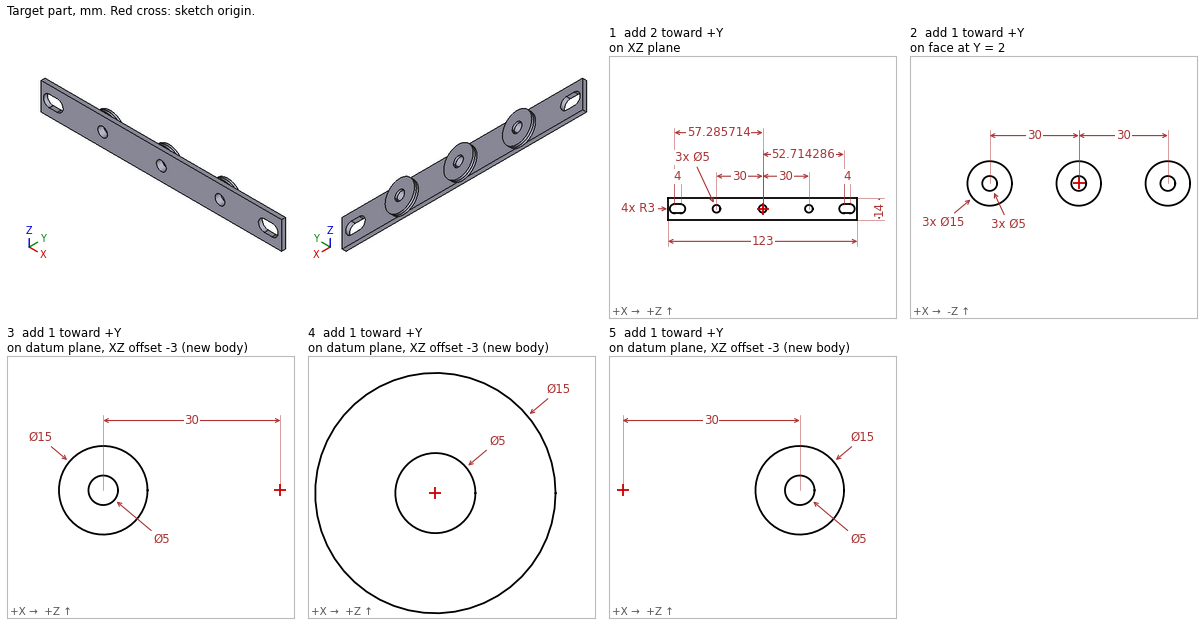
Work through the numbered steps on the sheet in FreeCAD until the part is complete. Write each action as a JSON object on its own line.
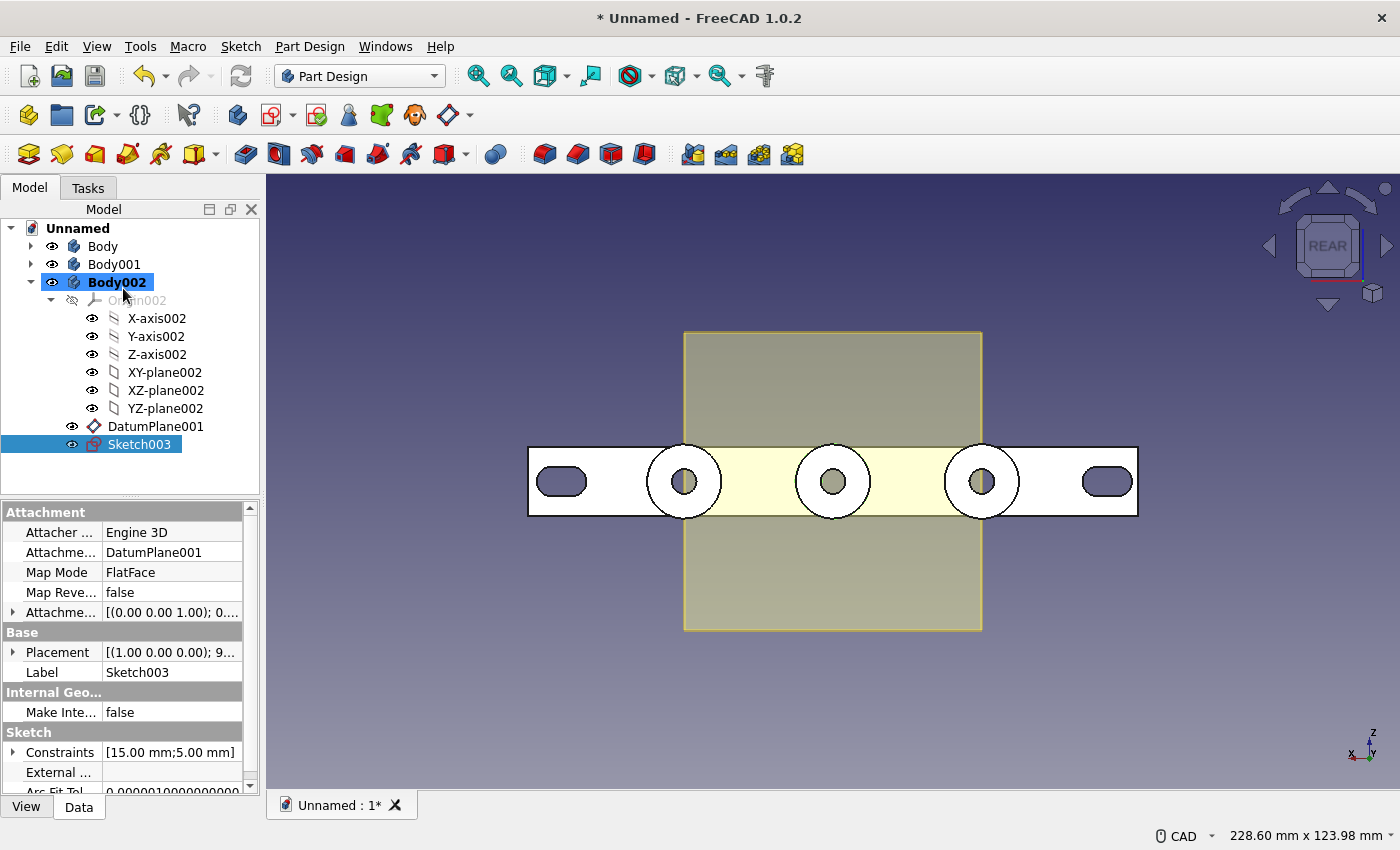
{"action": "left_click", "coordinate": [29, 154]}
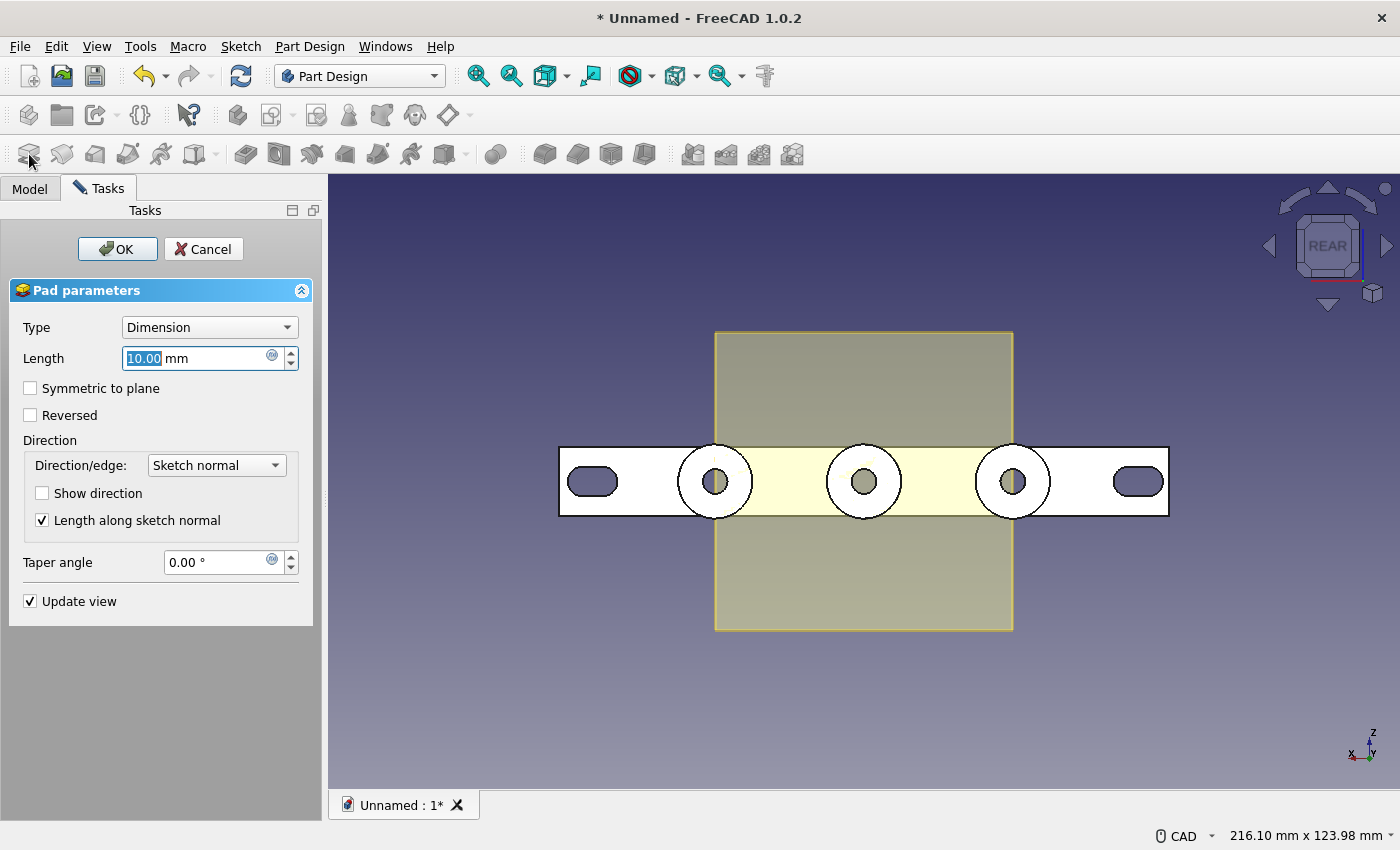
{"action": "type", "text": "1"}
{"action": "key", "text": "Tab"}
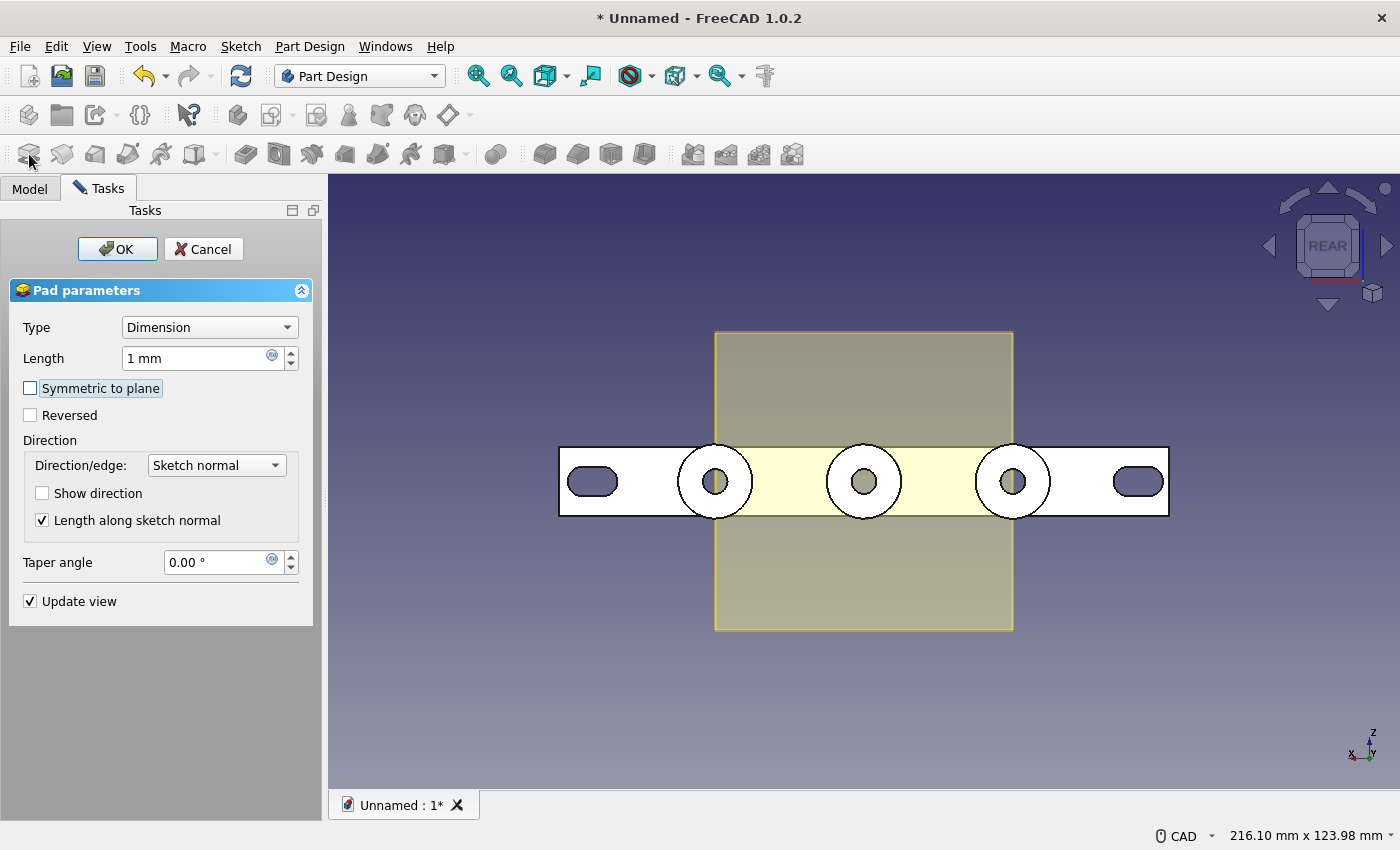
{"action": "left_click", "coordinate": [31, 415]}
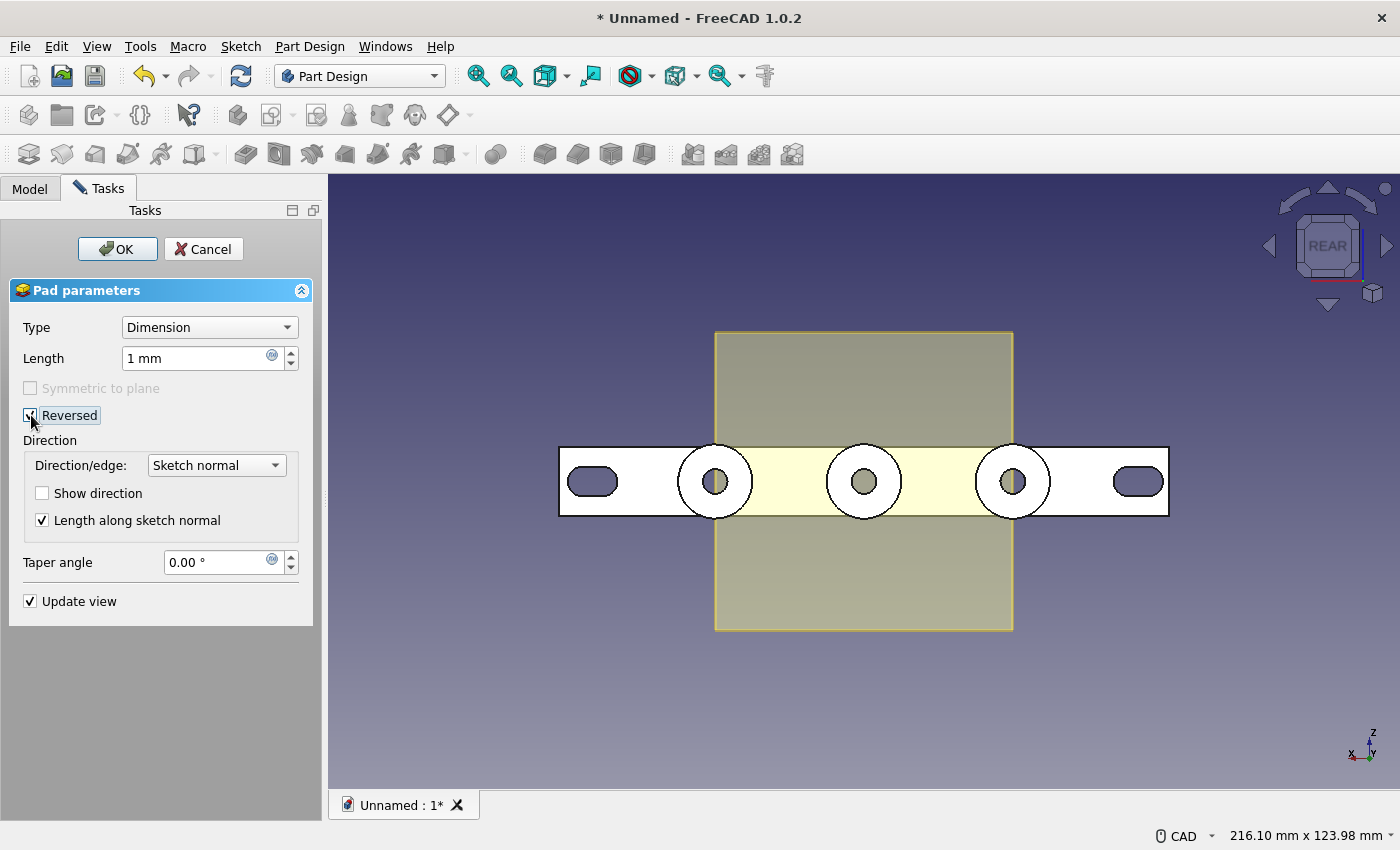
{"action": "left_click", "coordinate": [118, 249]}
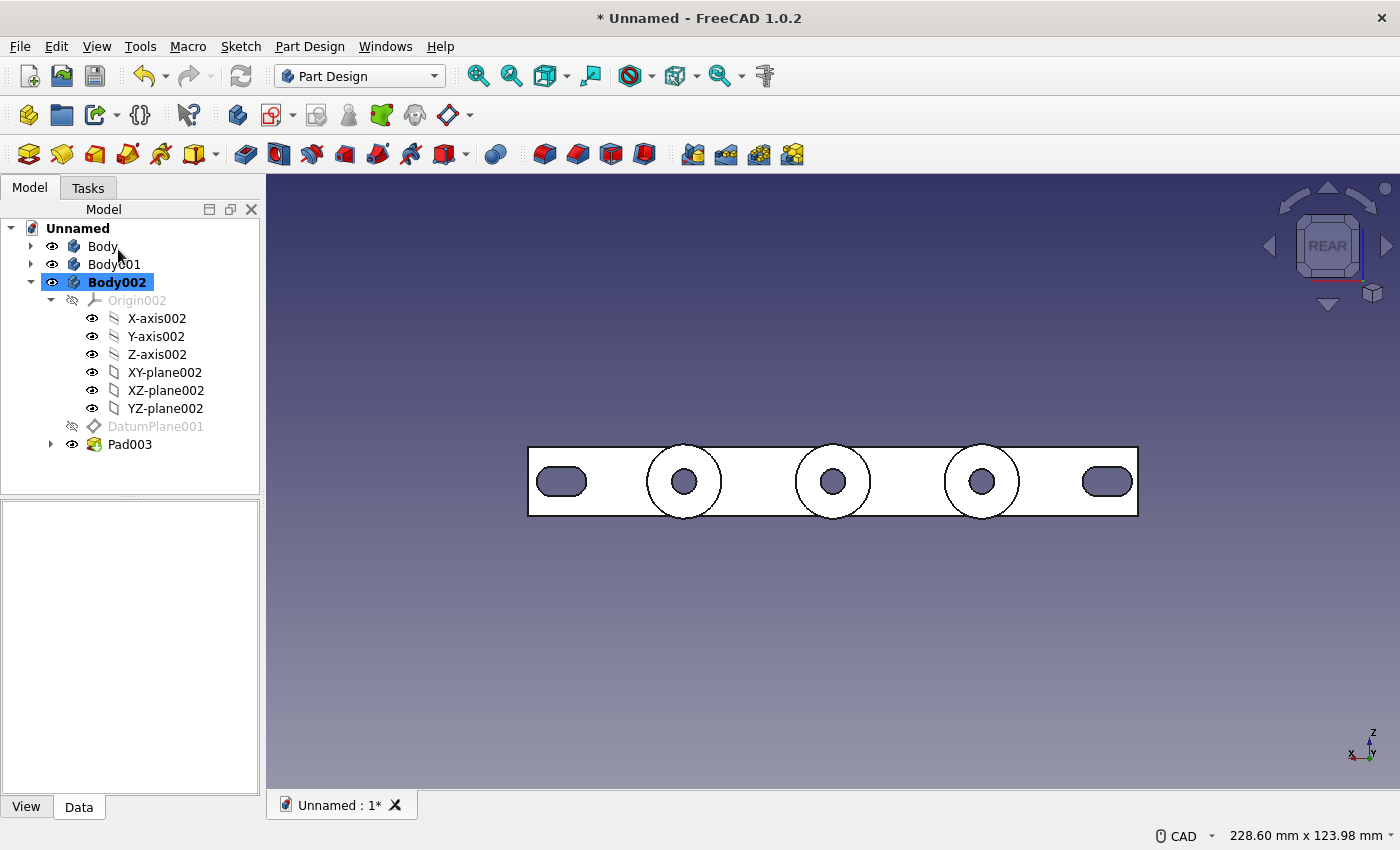
{"action": "left_click", "coordinate": [479, 76]}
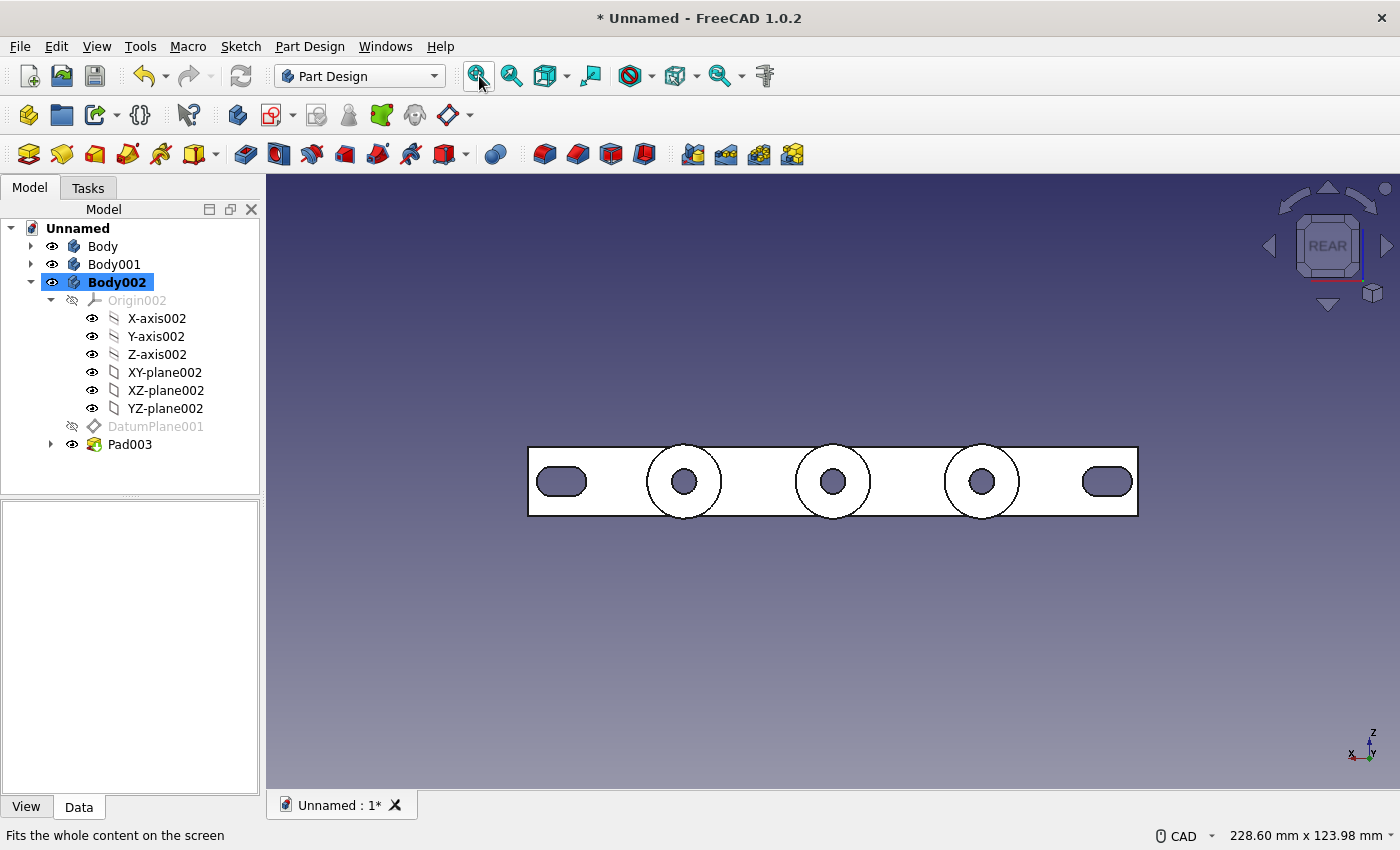
{"action": "left_click", "coordinate": [238, 116]}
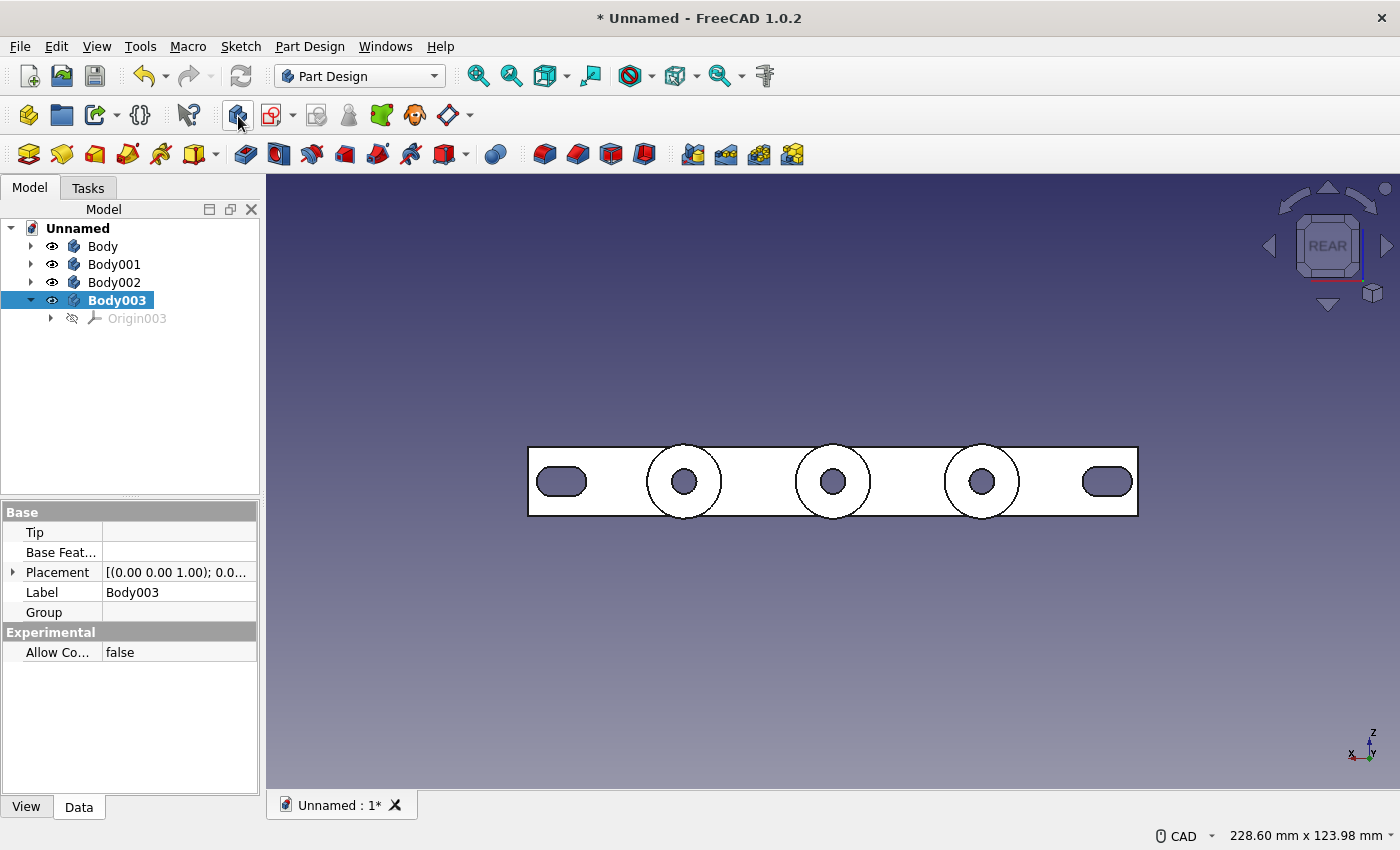
{"action": "left_click", "coordinate": [51, 318]}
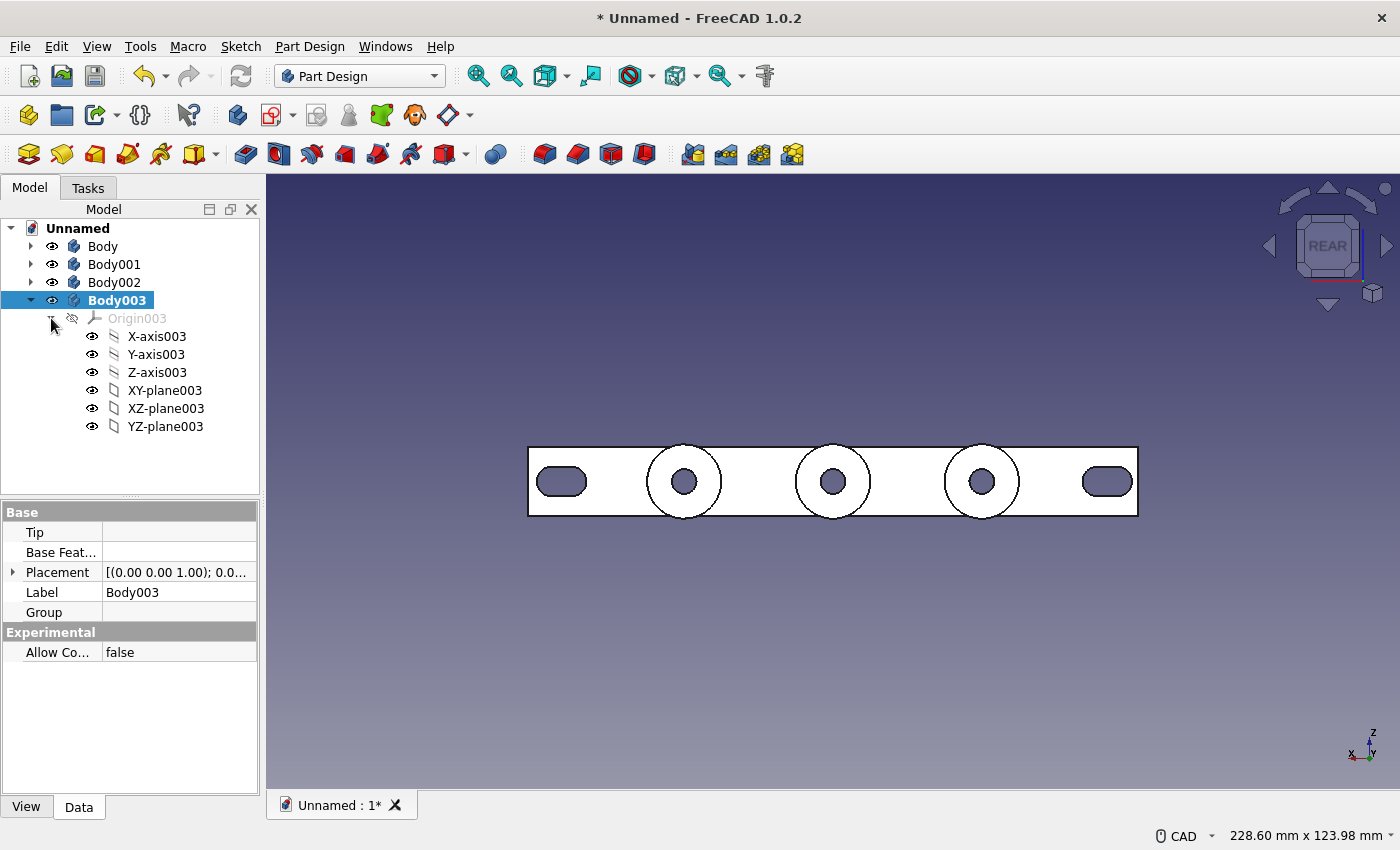
{"action": "left_click", "coordinate": [137, 408]}